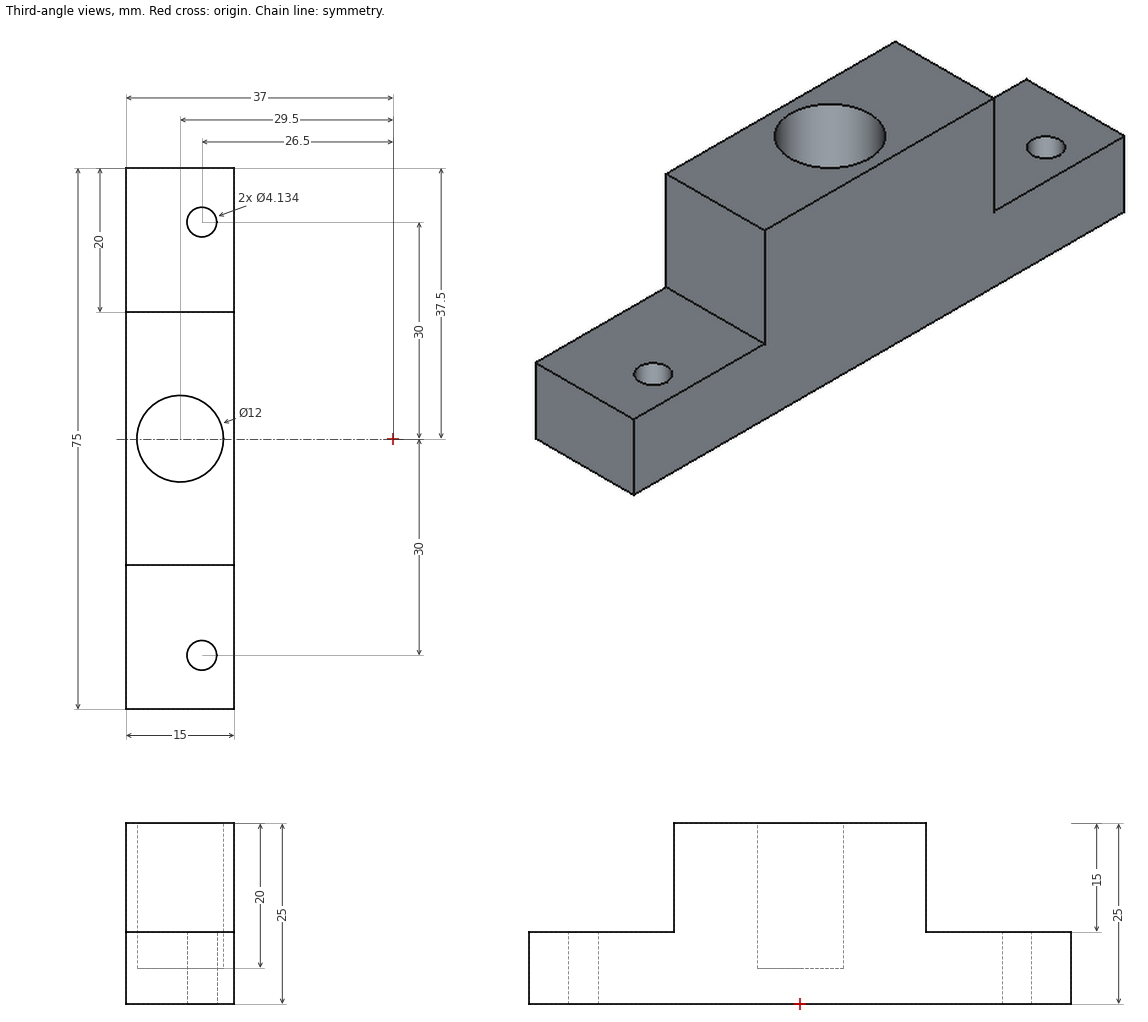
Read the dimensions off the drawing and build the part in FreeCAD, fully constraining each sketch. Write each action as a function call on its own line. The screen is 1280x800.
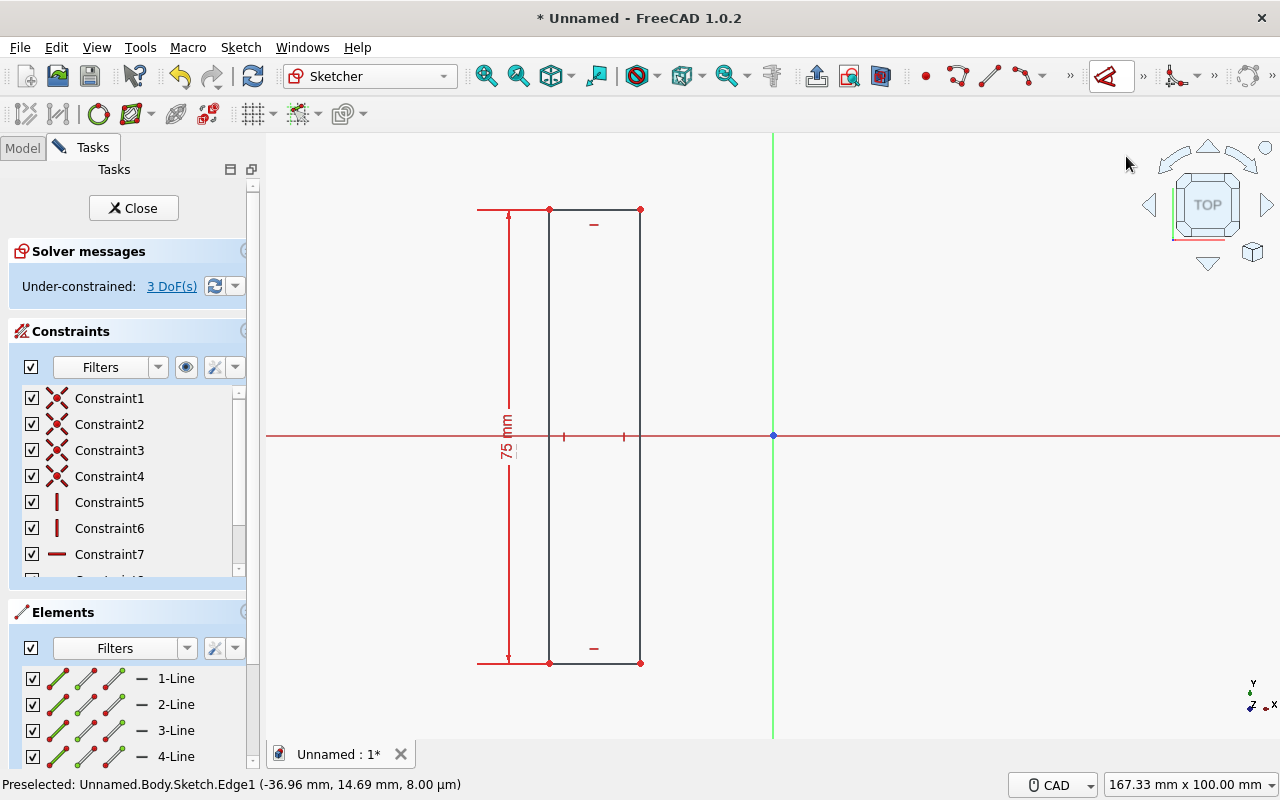
click(576, 664)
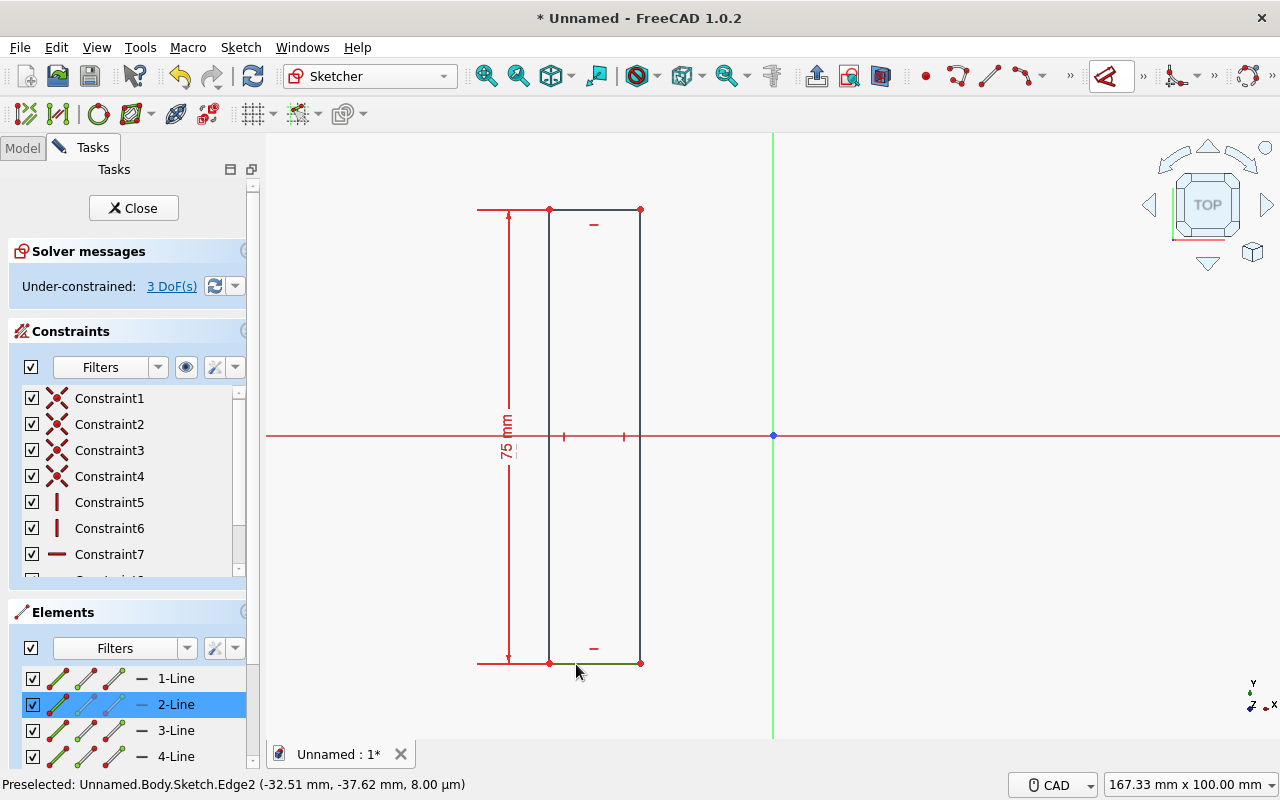
key(l)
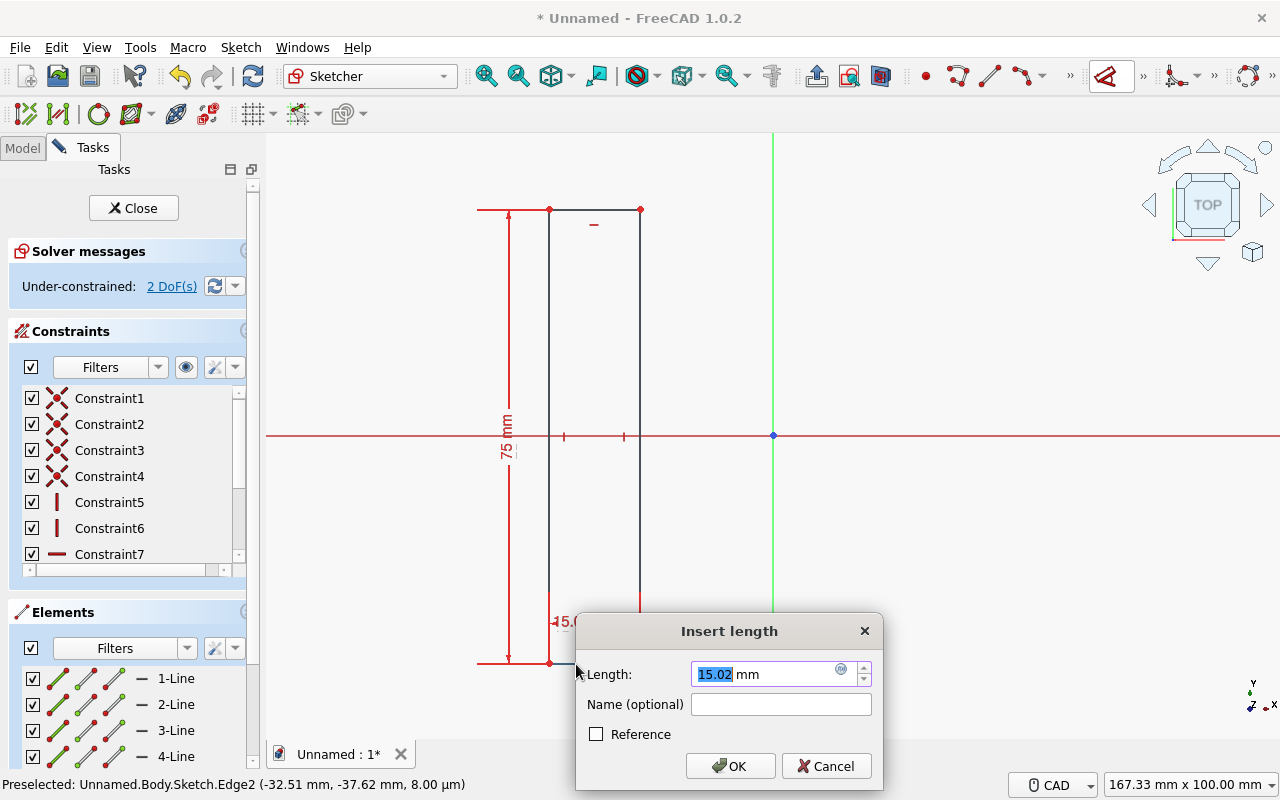
text(15)
key(Return)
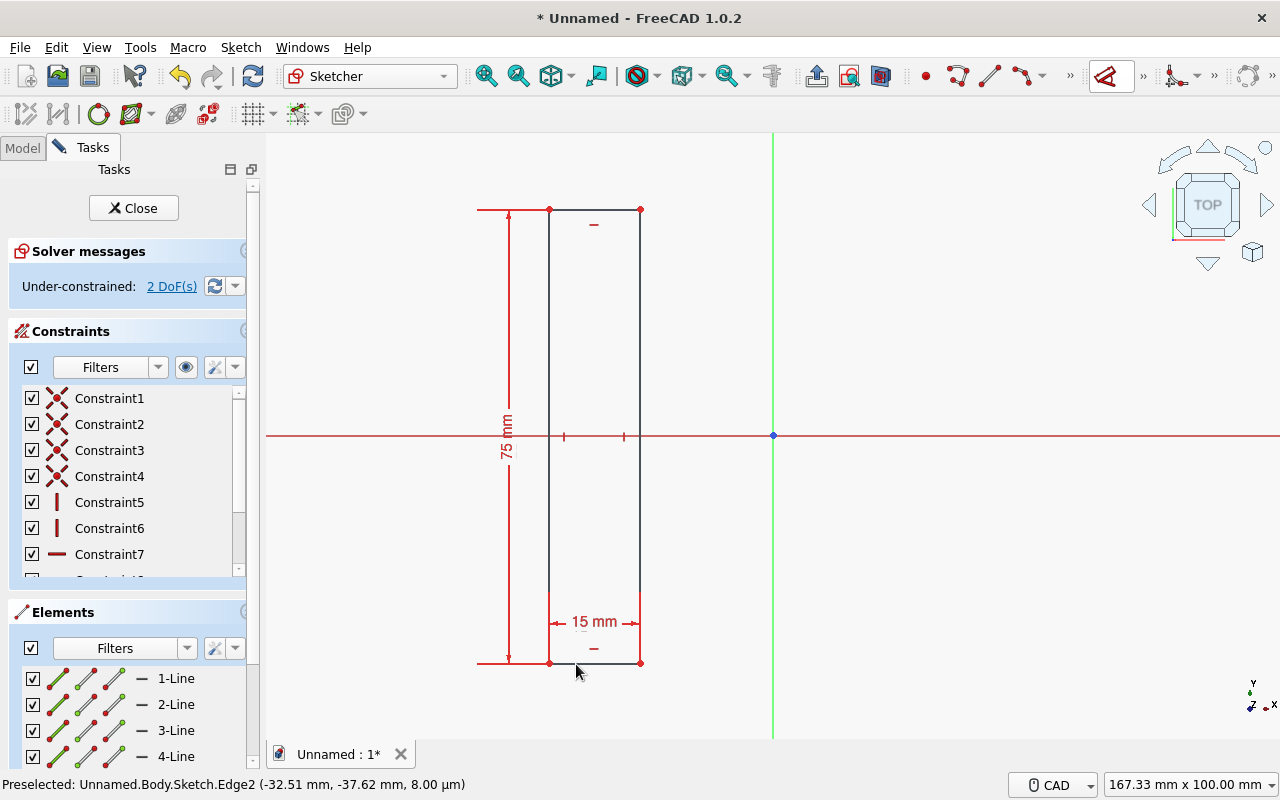
click(549, 210)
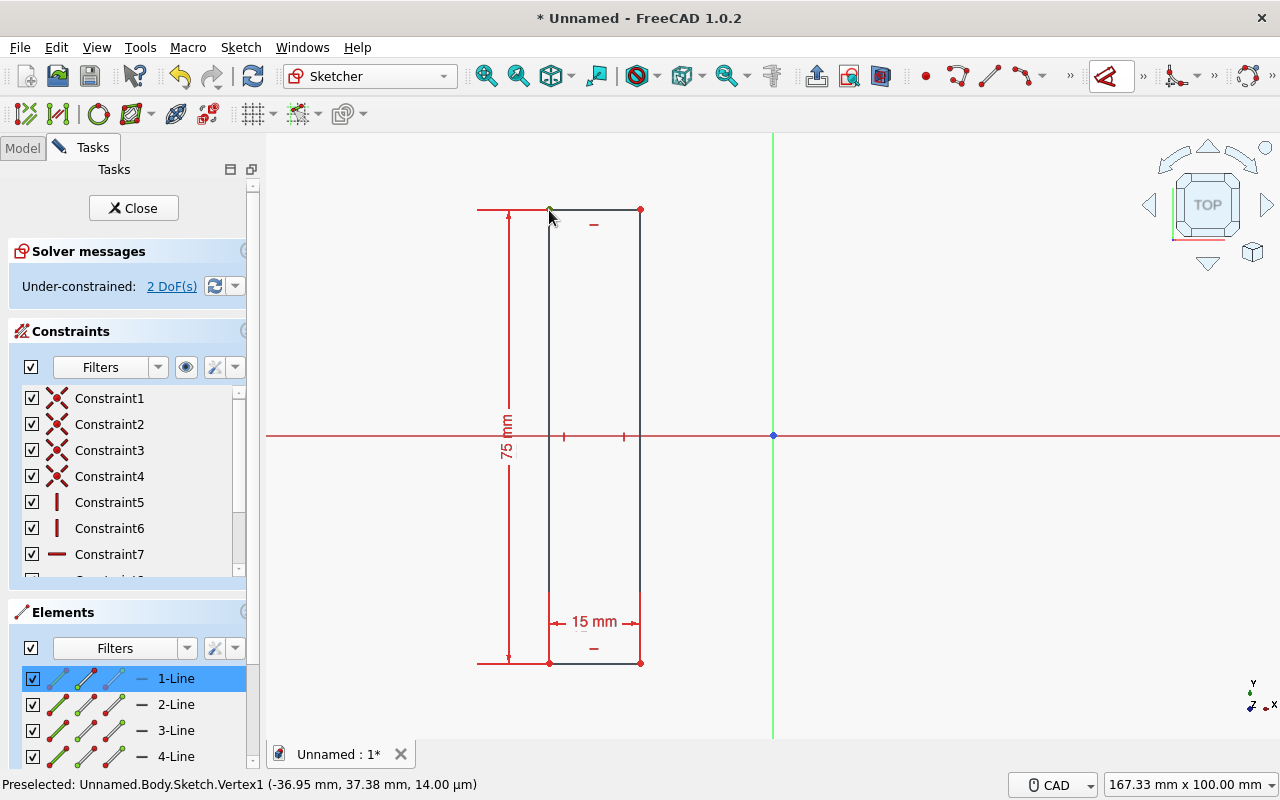
click(1128, 76)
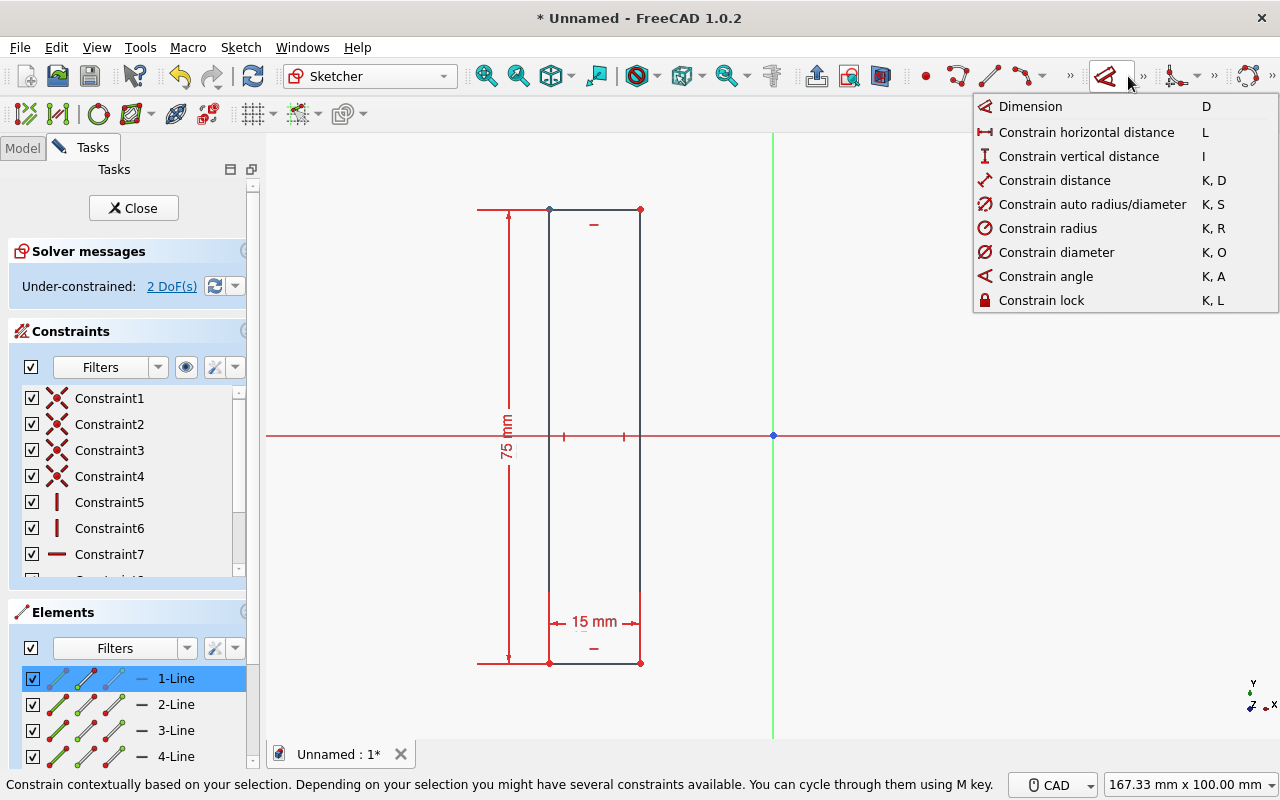
click(1126, 132)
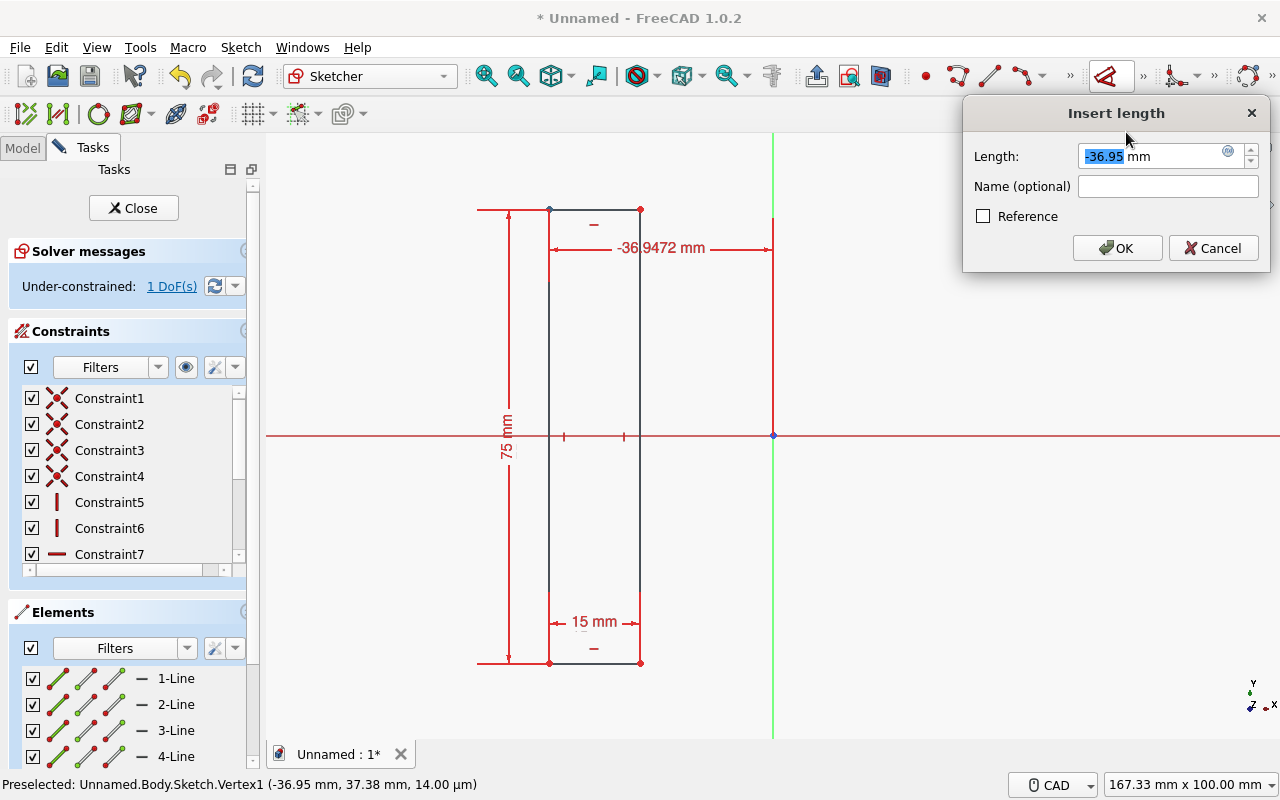
text(-37)
key(Return)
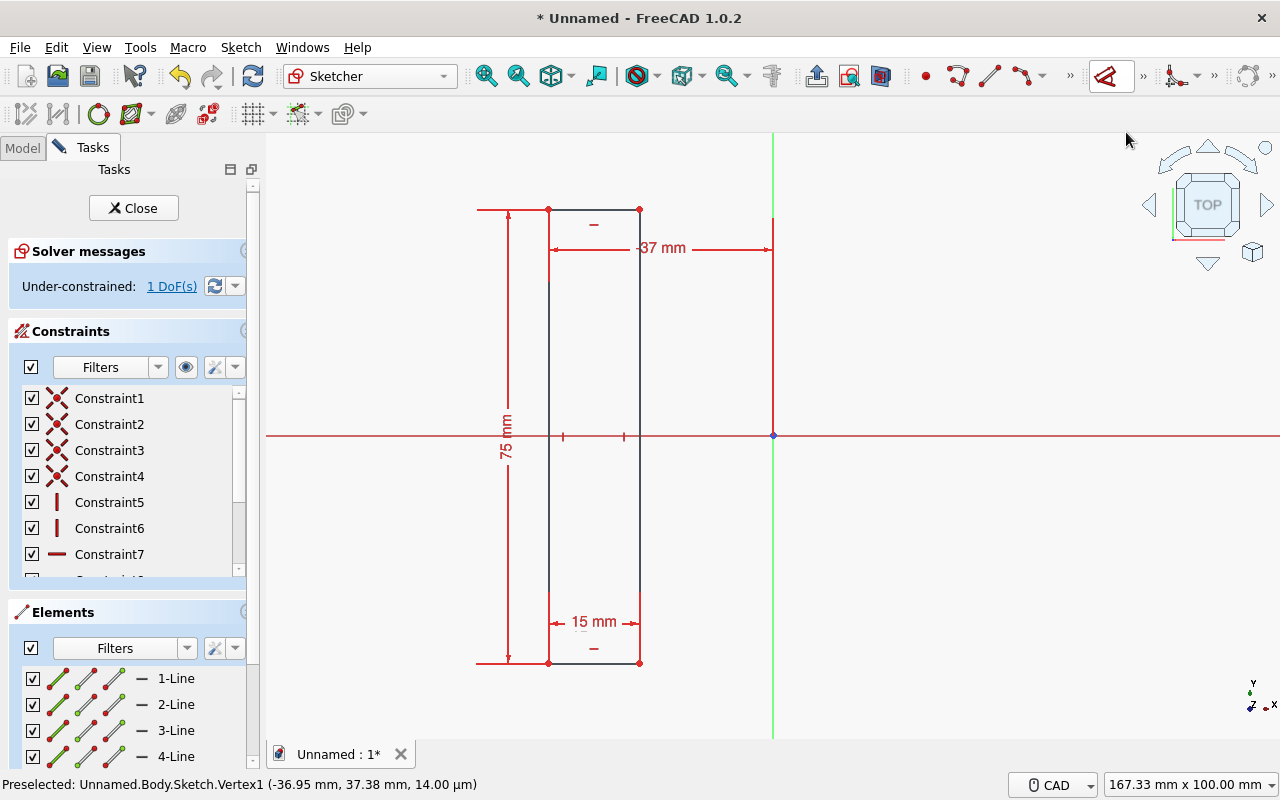
click(549, 210)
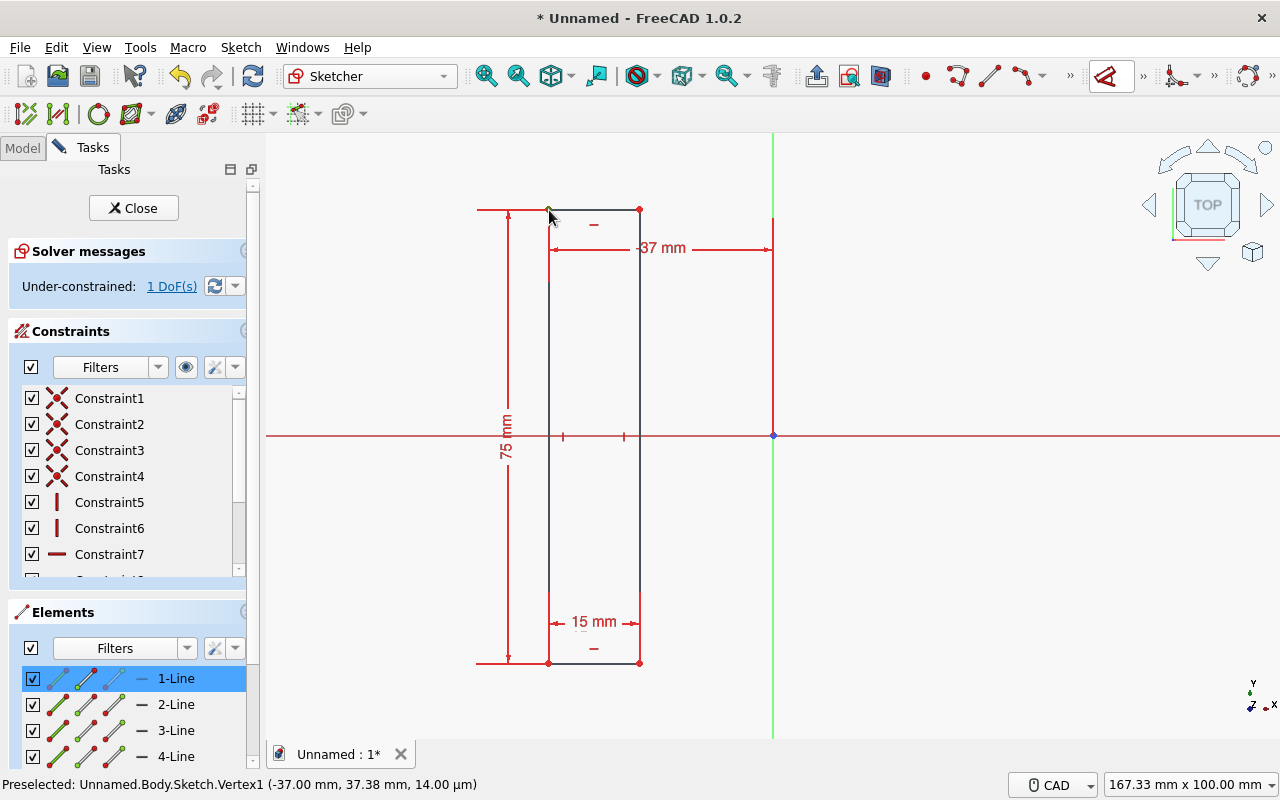
key(i)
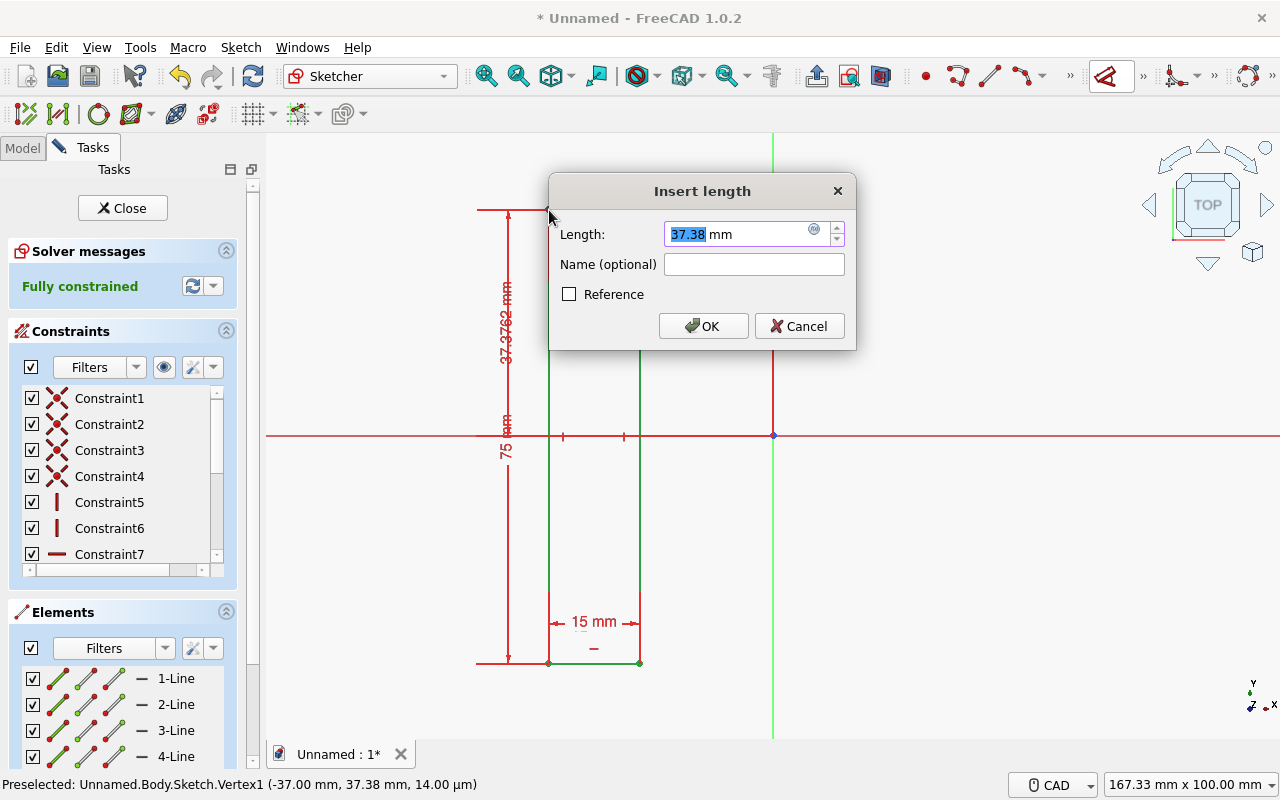
text(37.5)
key(Return)